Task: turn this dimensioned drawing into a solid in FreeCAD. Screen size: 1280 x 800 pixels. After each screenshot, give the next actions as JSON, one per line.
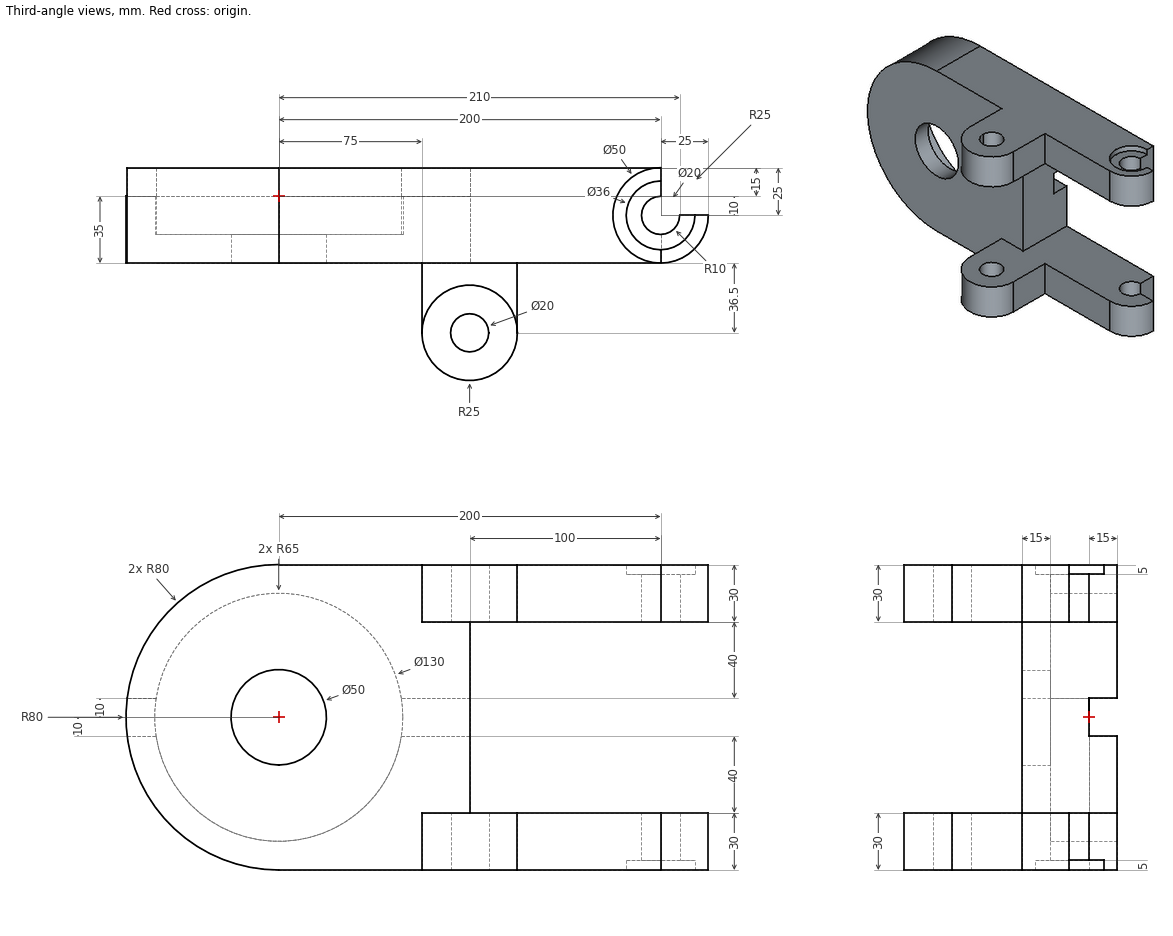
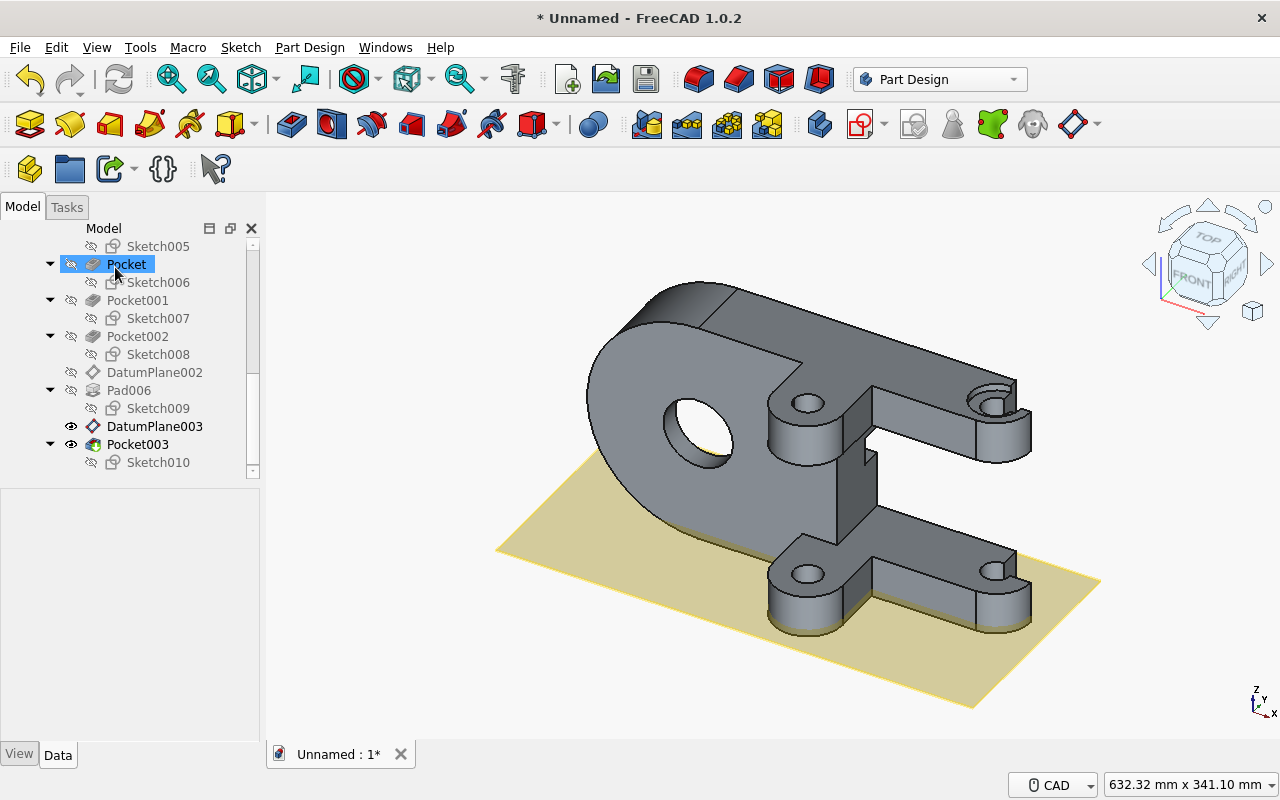
{"action": "left_click", "coordinate": [116, 426]}
{"action": "key", "text": "space"}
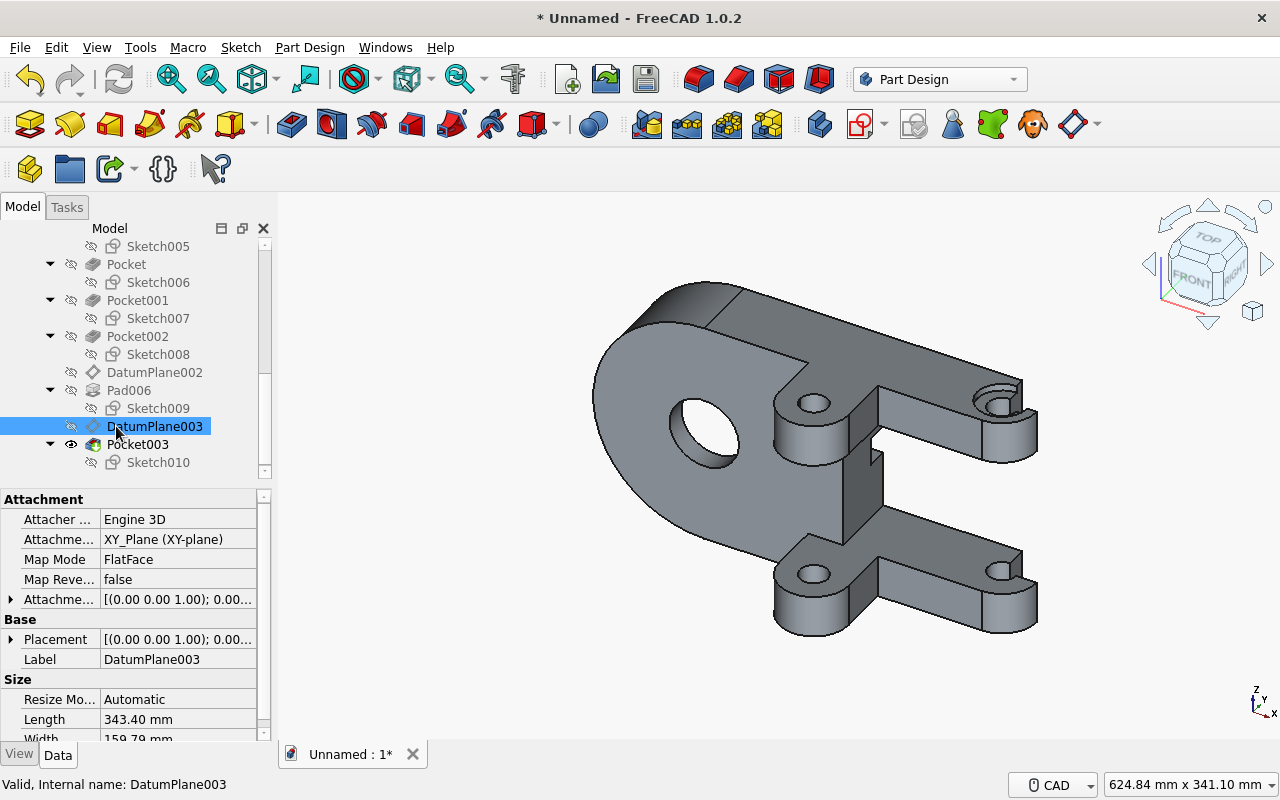
{"action": "key", "text": "0"}